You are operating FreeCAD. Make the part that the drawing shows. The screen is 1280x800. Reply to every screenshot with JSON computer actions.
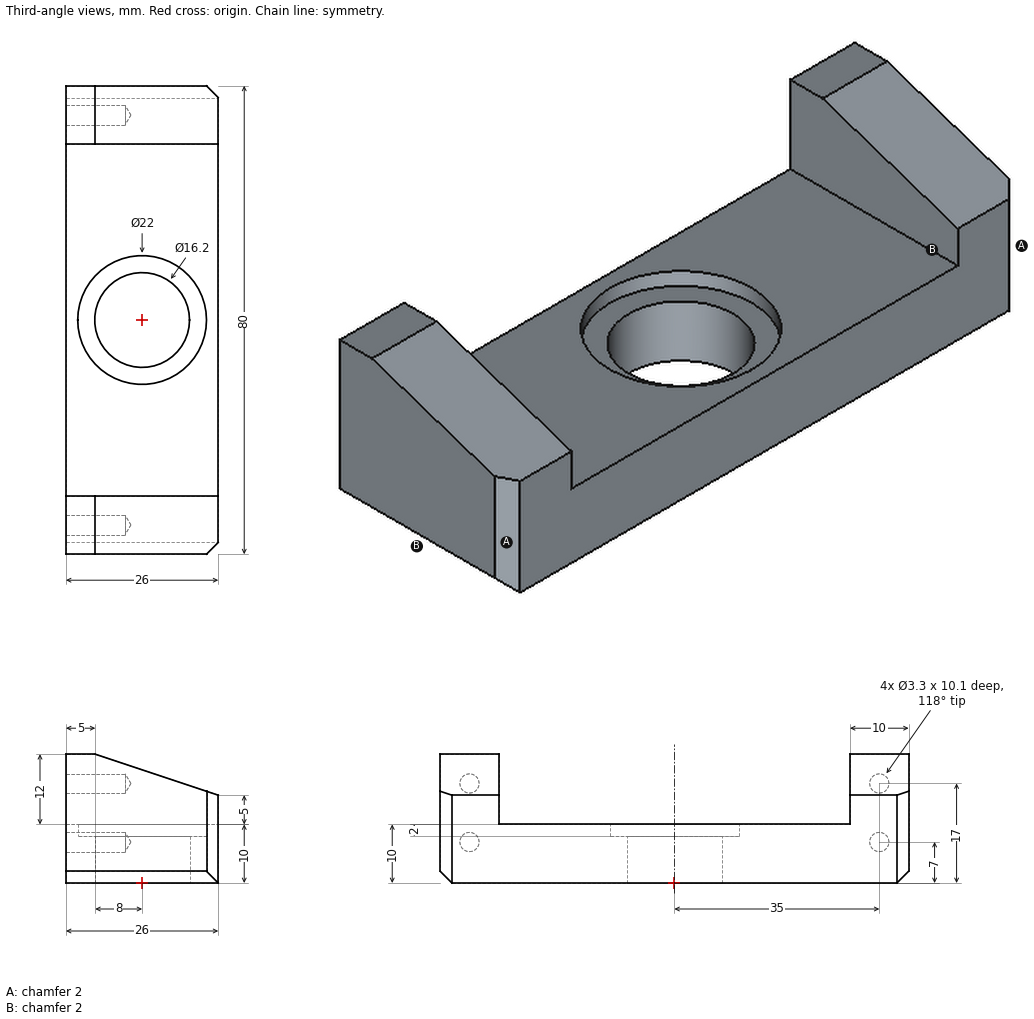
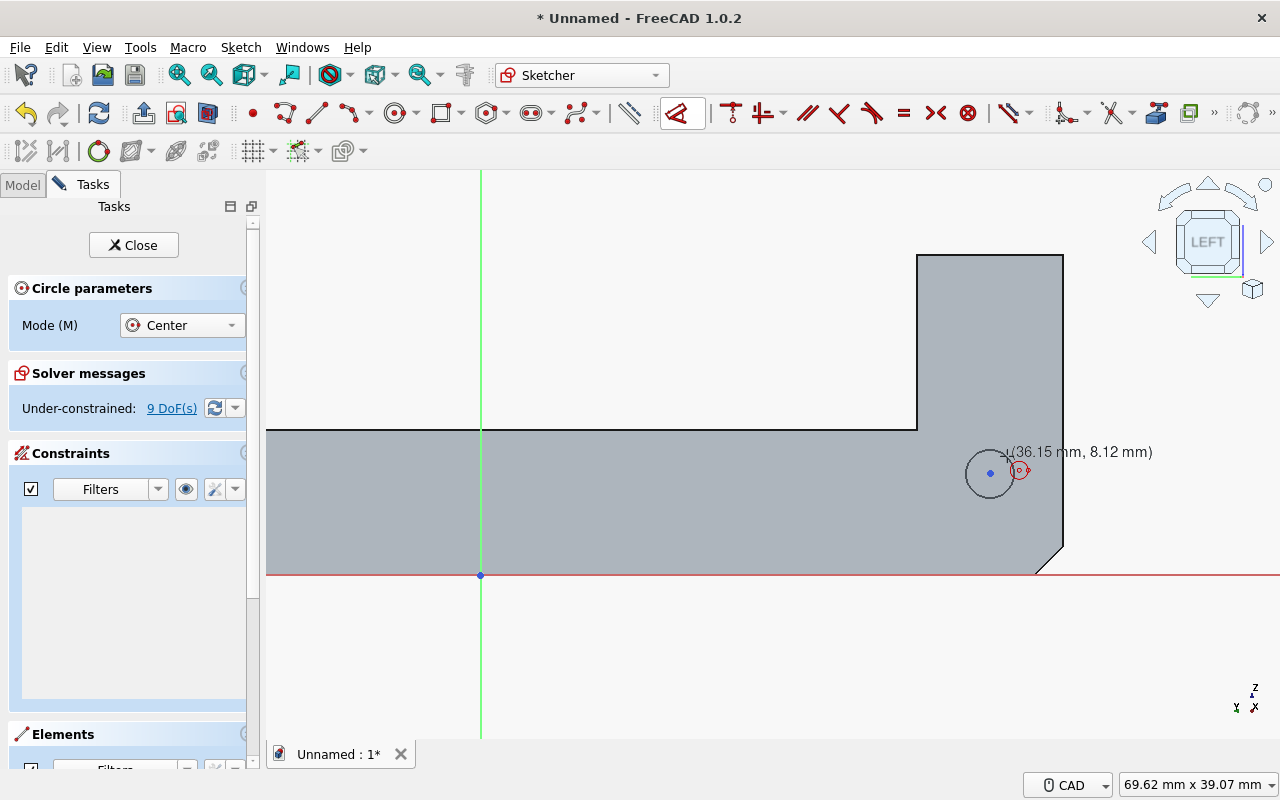
{"action": "left_click", "coordinate": [990, 328]}
{"action": "left_click", "coordinate": [1007, 311]}
{"action": "key", "text": "Escape"}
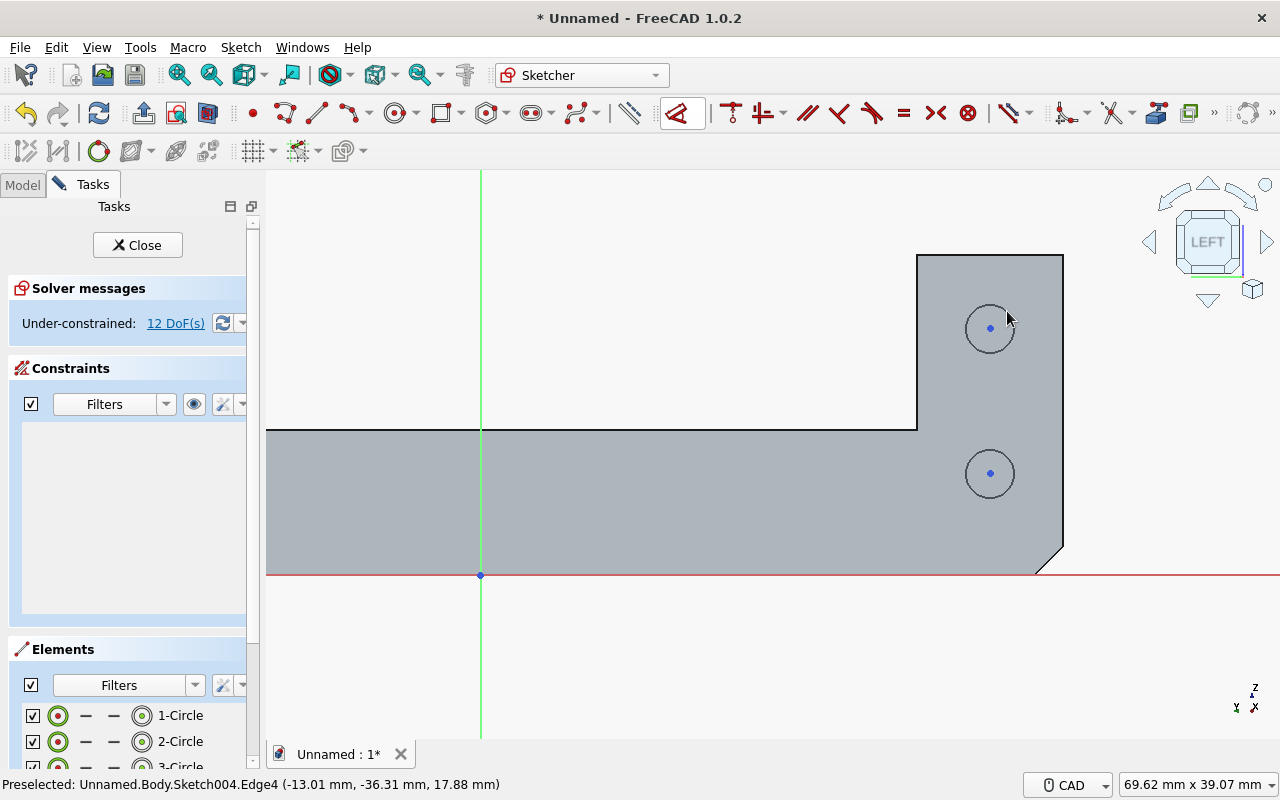
{"action": "scroll", "coordinate": [977, 473], "scroll_direction": "down", "scroll_amount": 3}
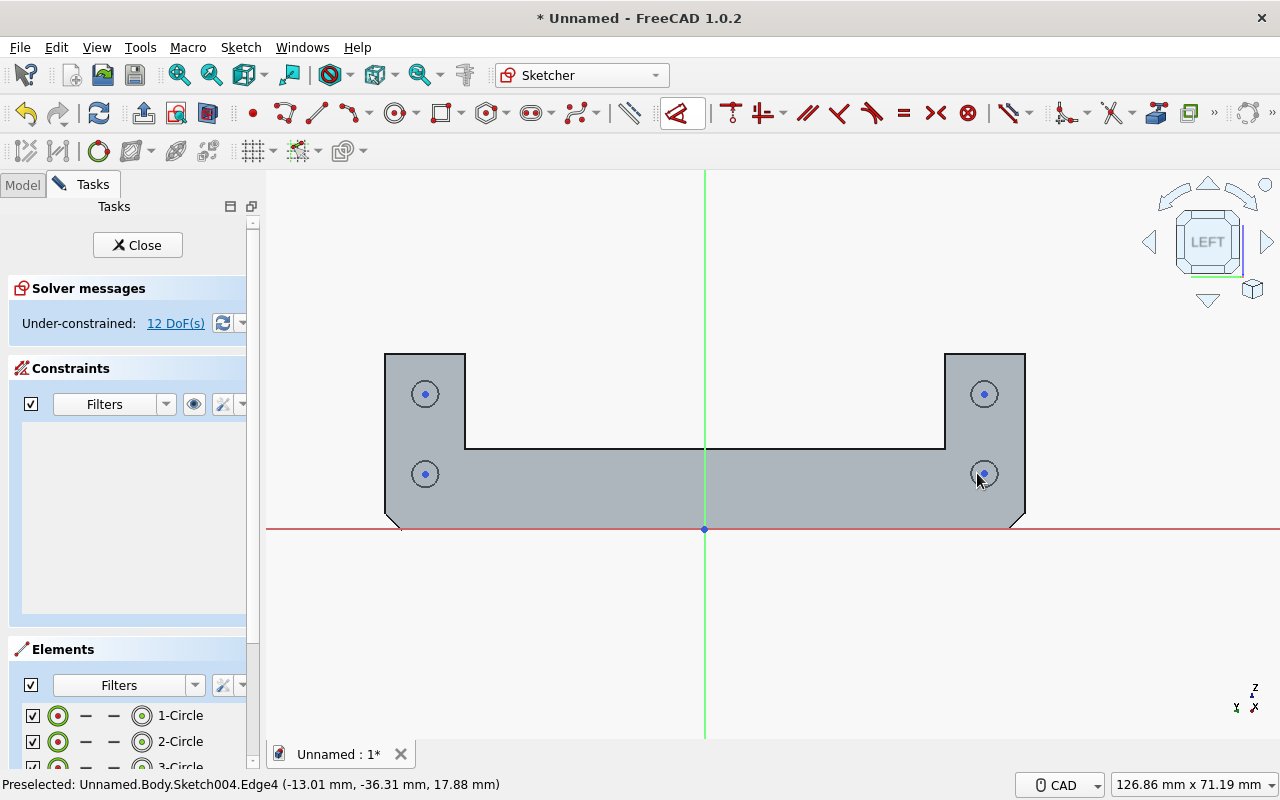
{"action": "left_click", "coordinate": [435, 385]}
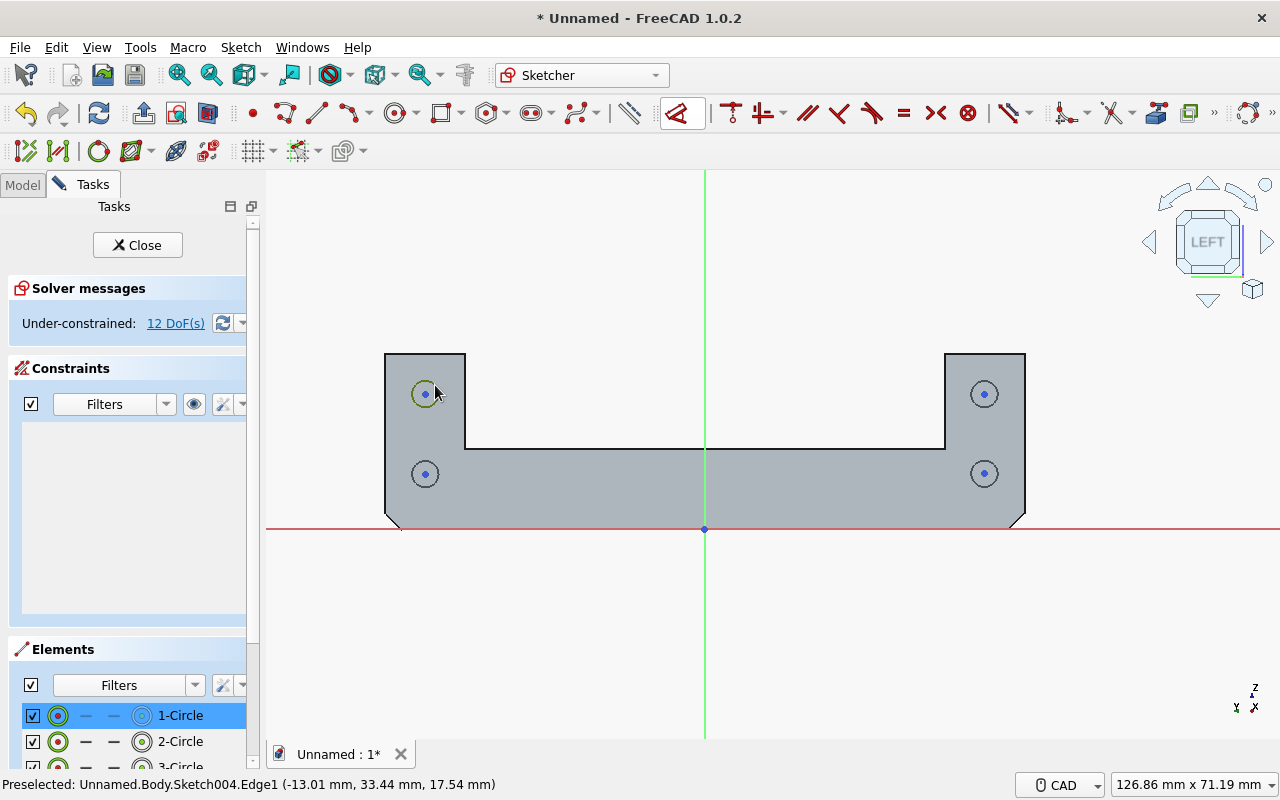
{"action": "left_click", "coordinate": [435, 465]}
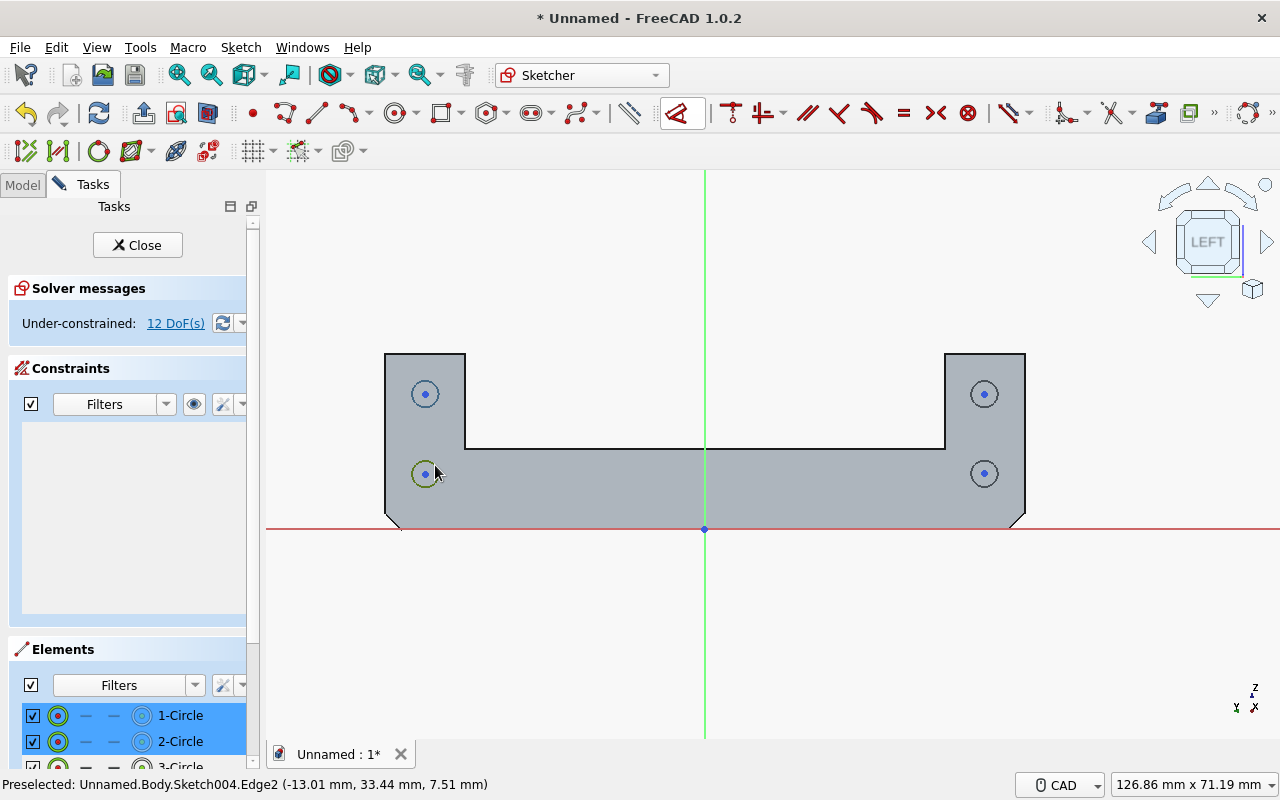
{"action": "left_click", "coordinate": [994, 464]}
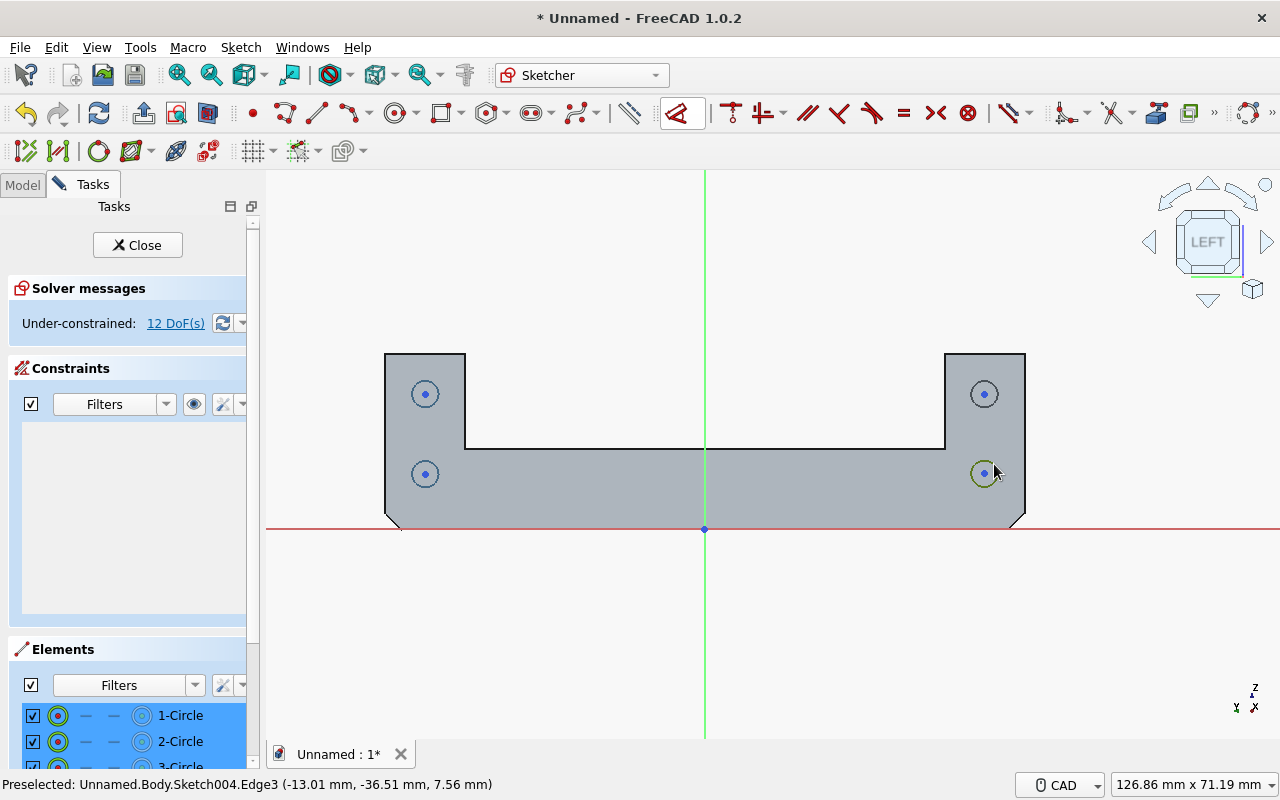
{"action": "left_click", "coordinate": [994, 385]}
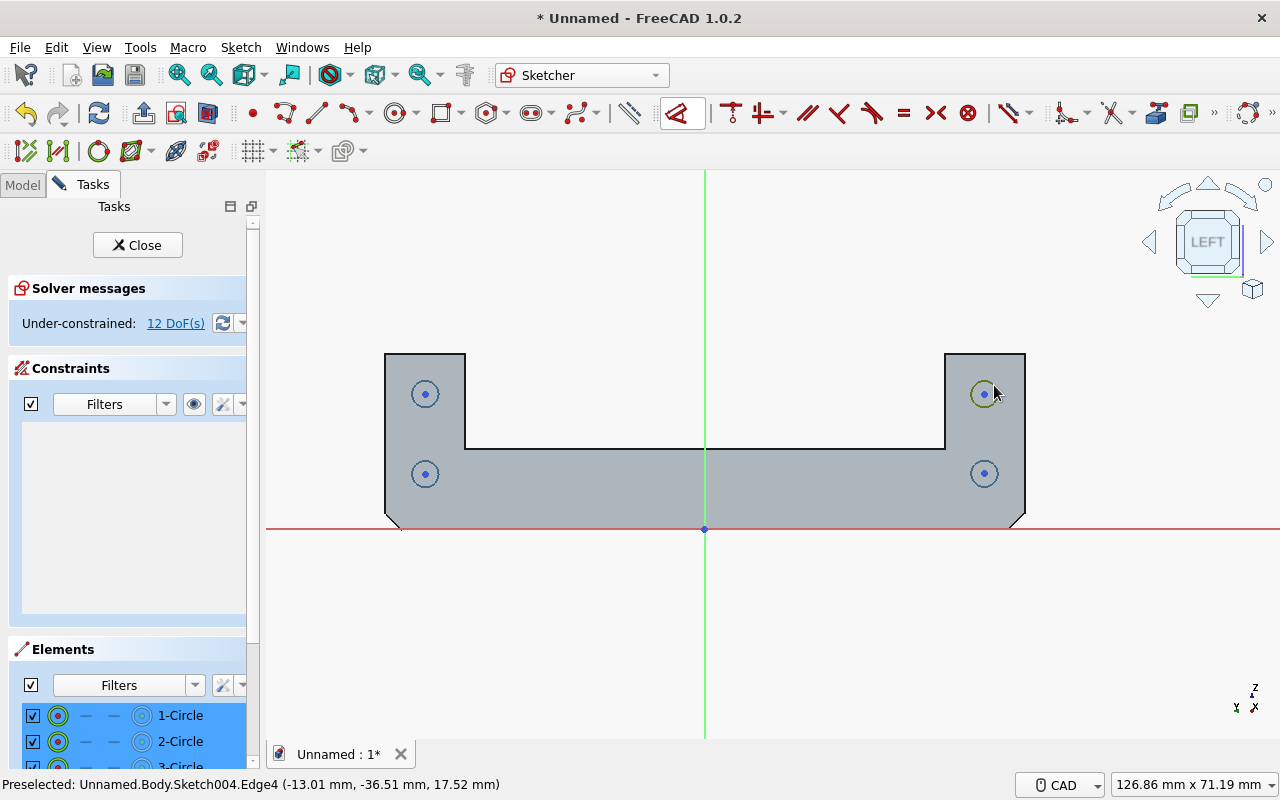
{"action": "left_click", "coordinate": [904, 114]}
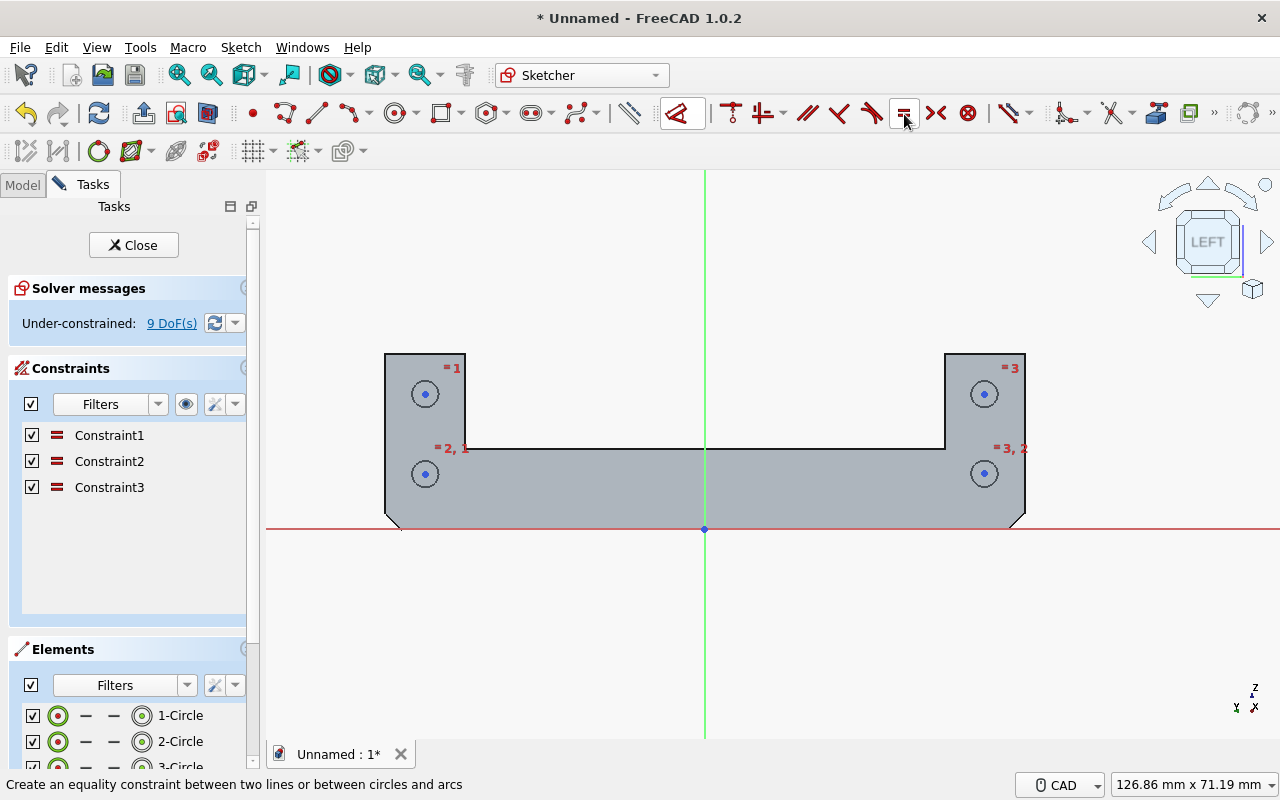
{"action": "left_click", "coordinate": [425, 474]}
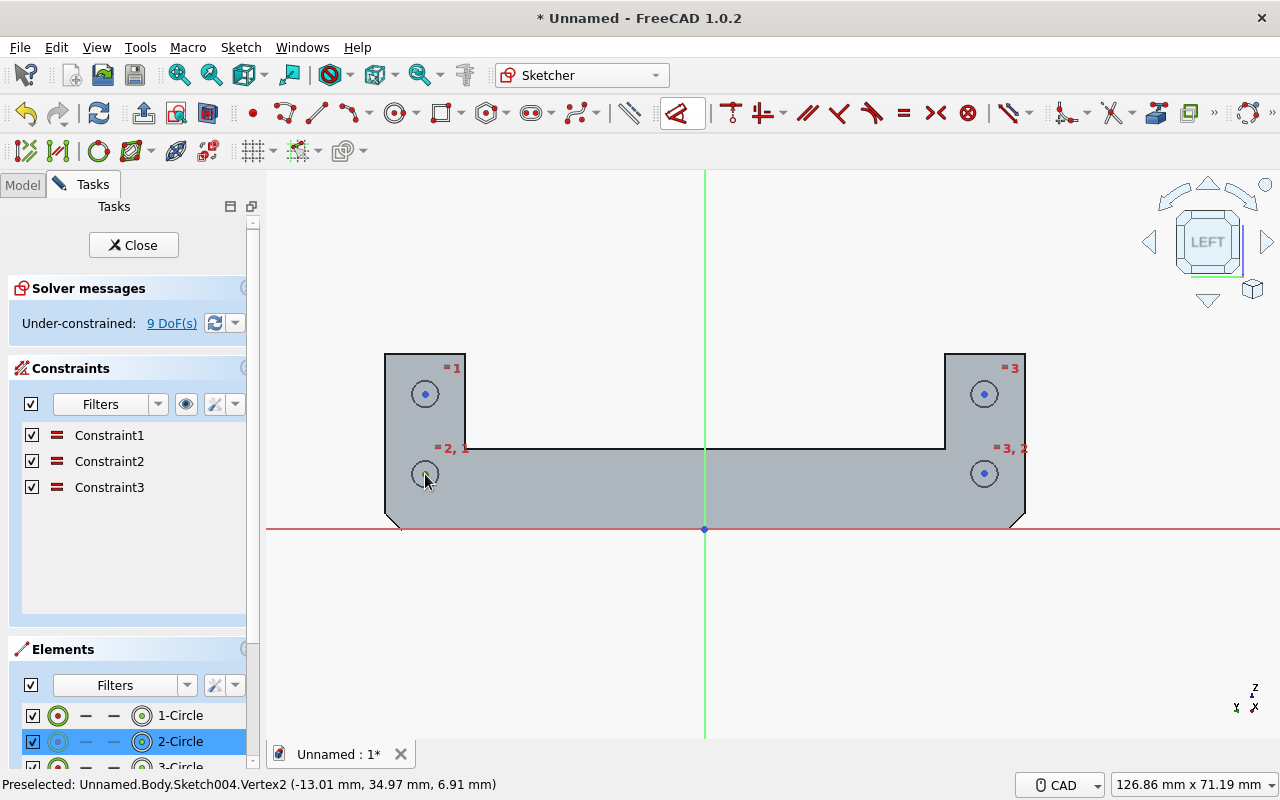
{"action": "left_click", "coordinate": [984, 474]}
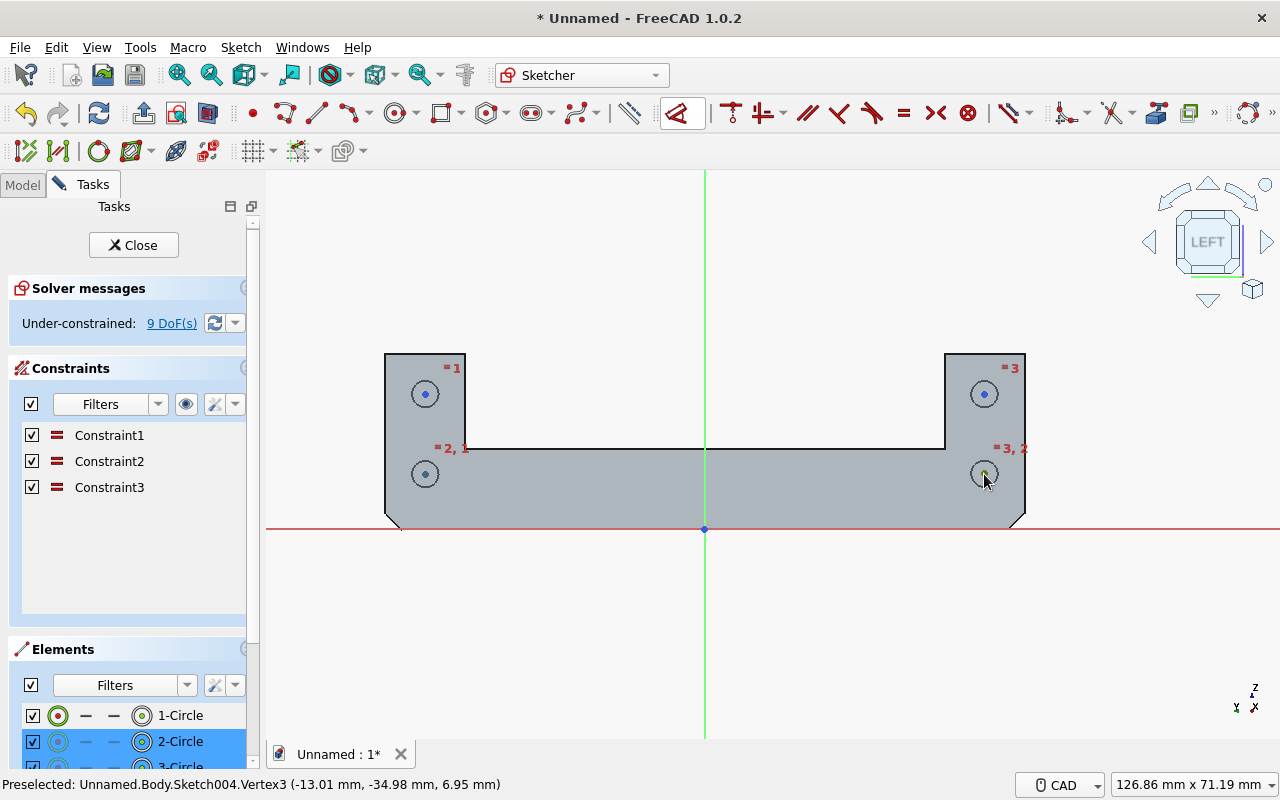
{"action": "left_click", "coordinate": [705, 674]}